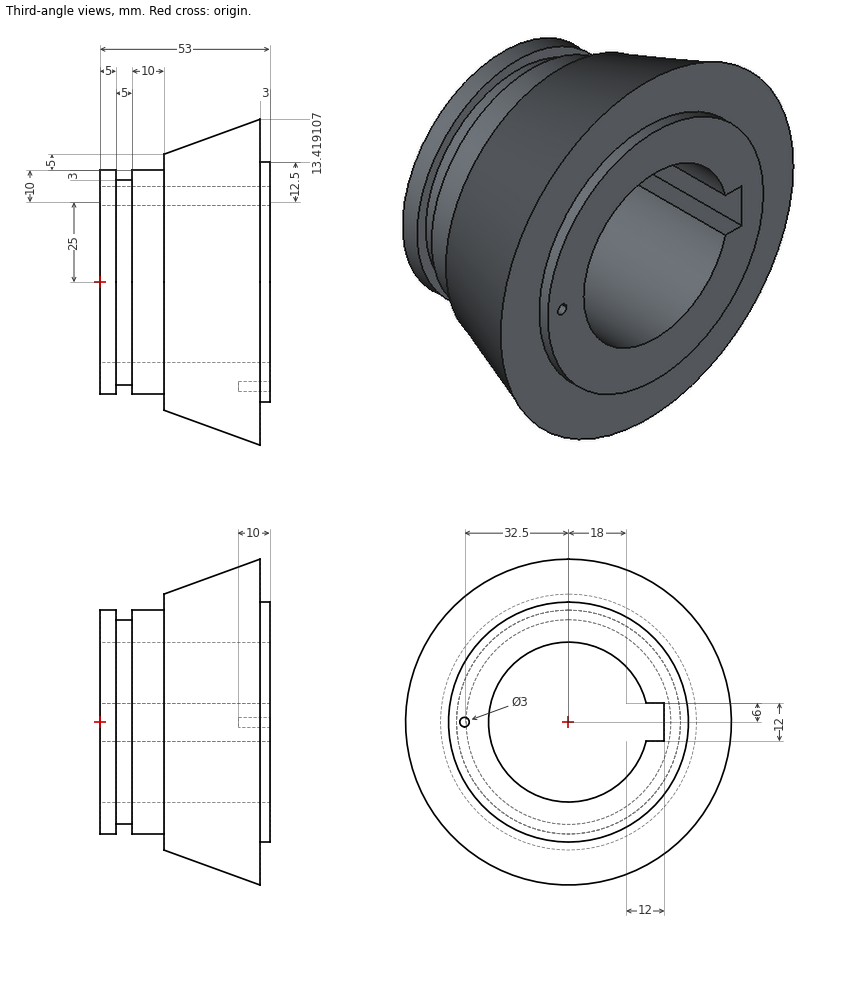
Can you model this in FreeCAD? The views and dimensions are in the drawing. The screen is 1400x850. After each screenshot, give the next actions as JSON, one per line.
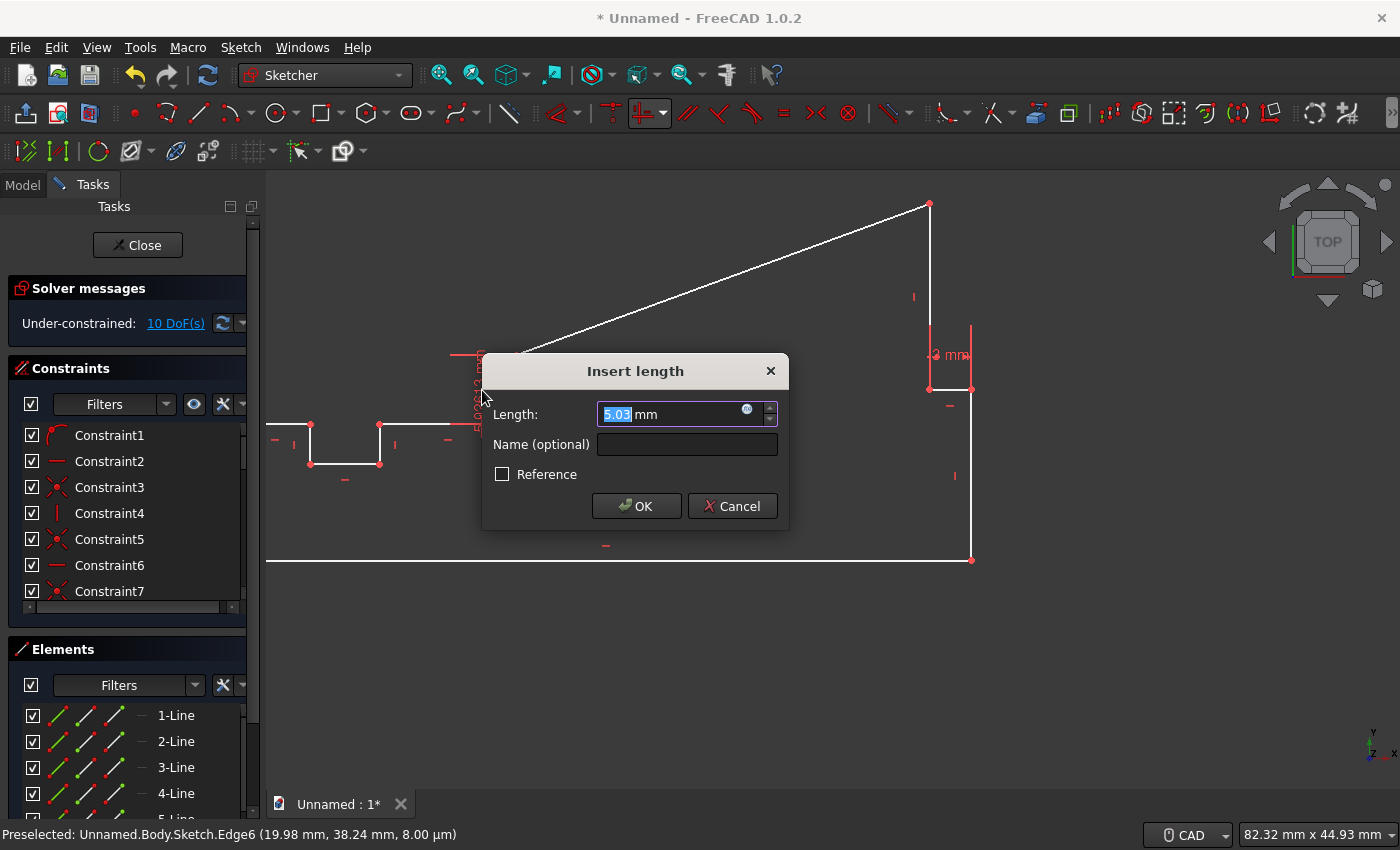
{"action": "type", "text": "5"}
{"action": "key", "text": "Return"}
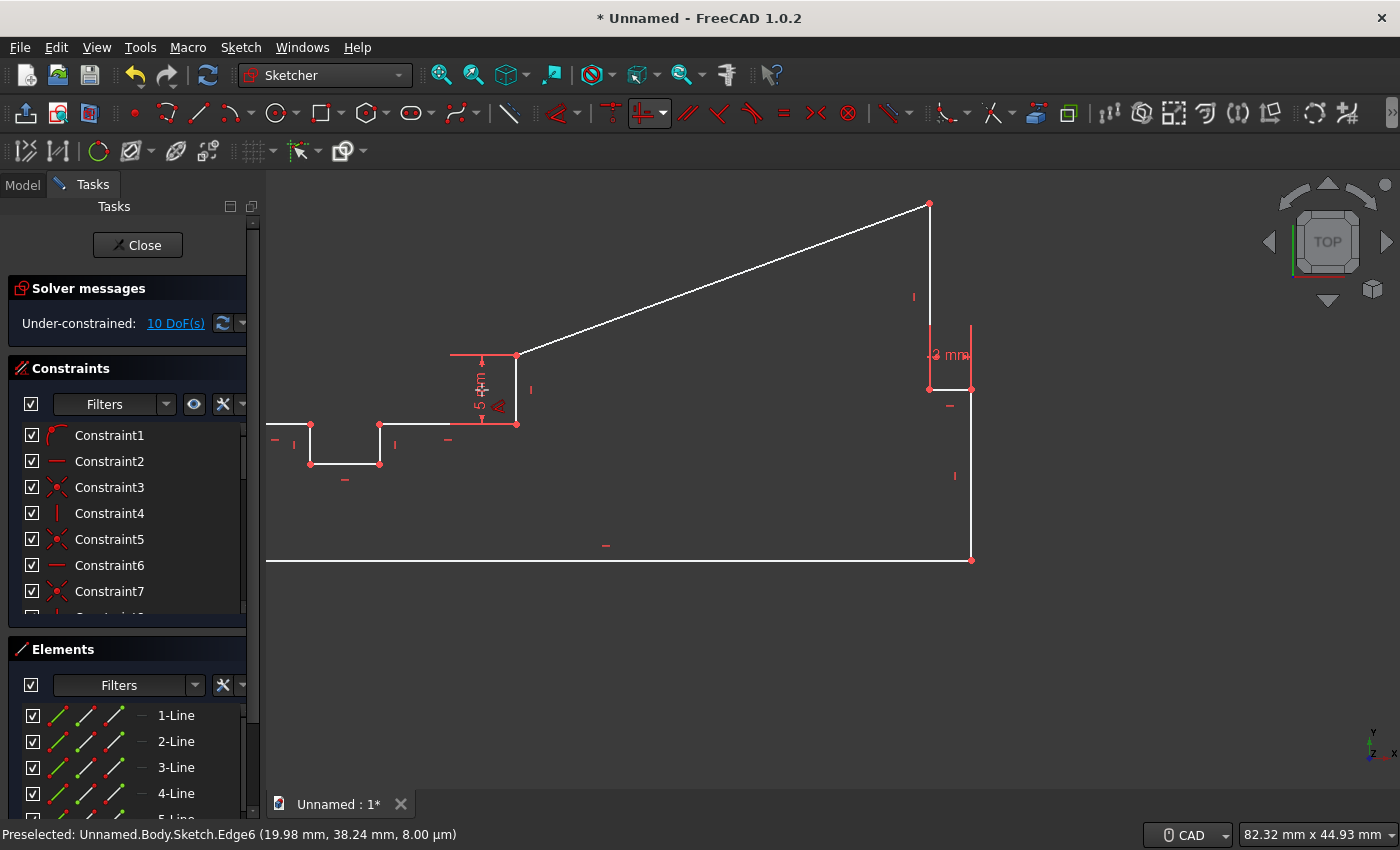
{"action": "left_click", "coordinate": [380, 436]}
{"action": "left_click", "coordinate": [346, 444]}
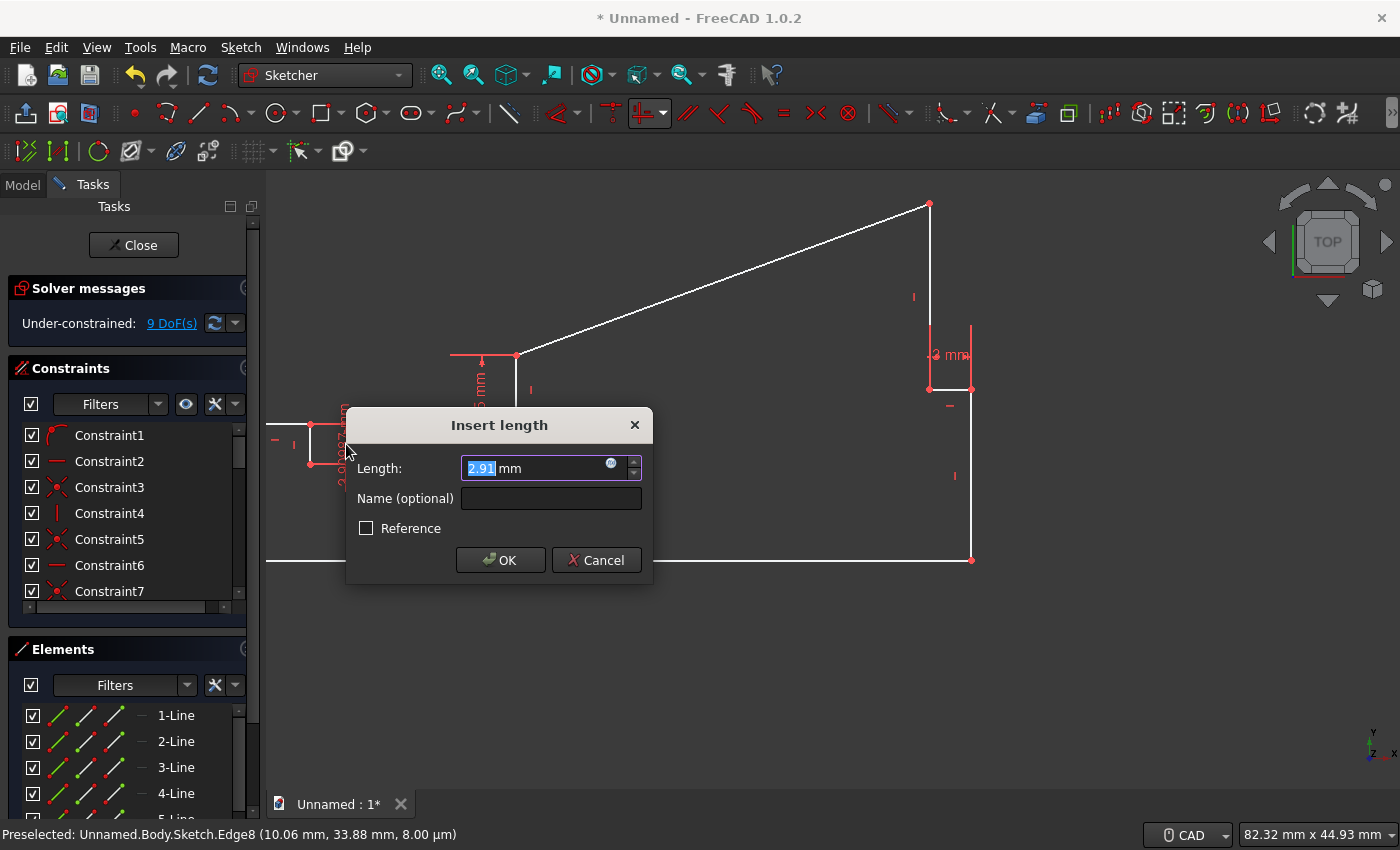
{"action": "type", "text": "3"}
{"action": "key", "text": "Return"}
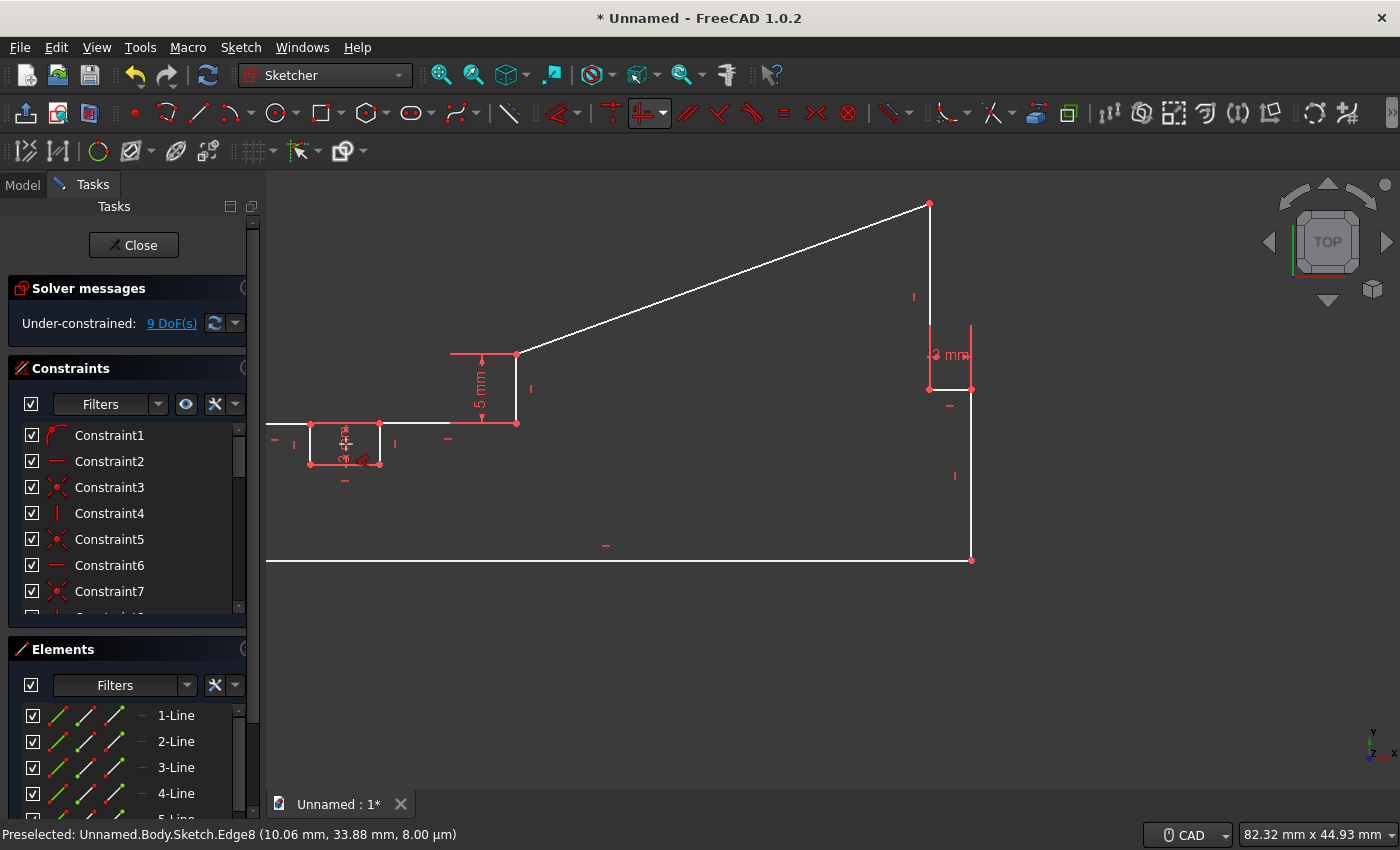
{"action": "left_click", "coordinate": [359, 465]}
{"action": "left_click", "coordinate": [345, 499]}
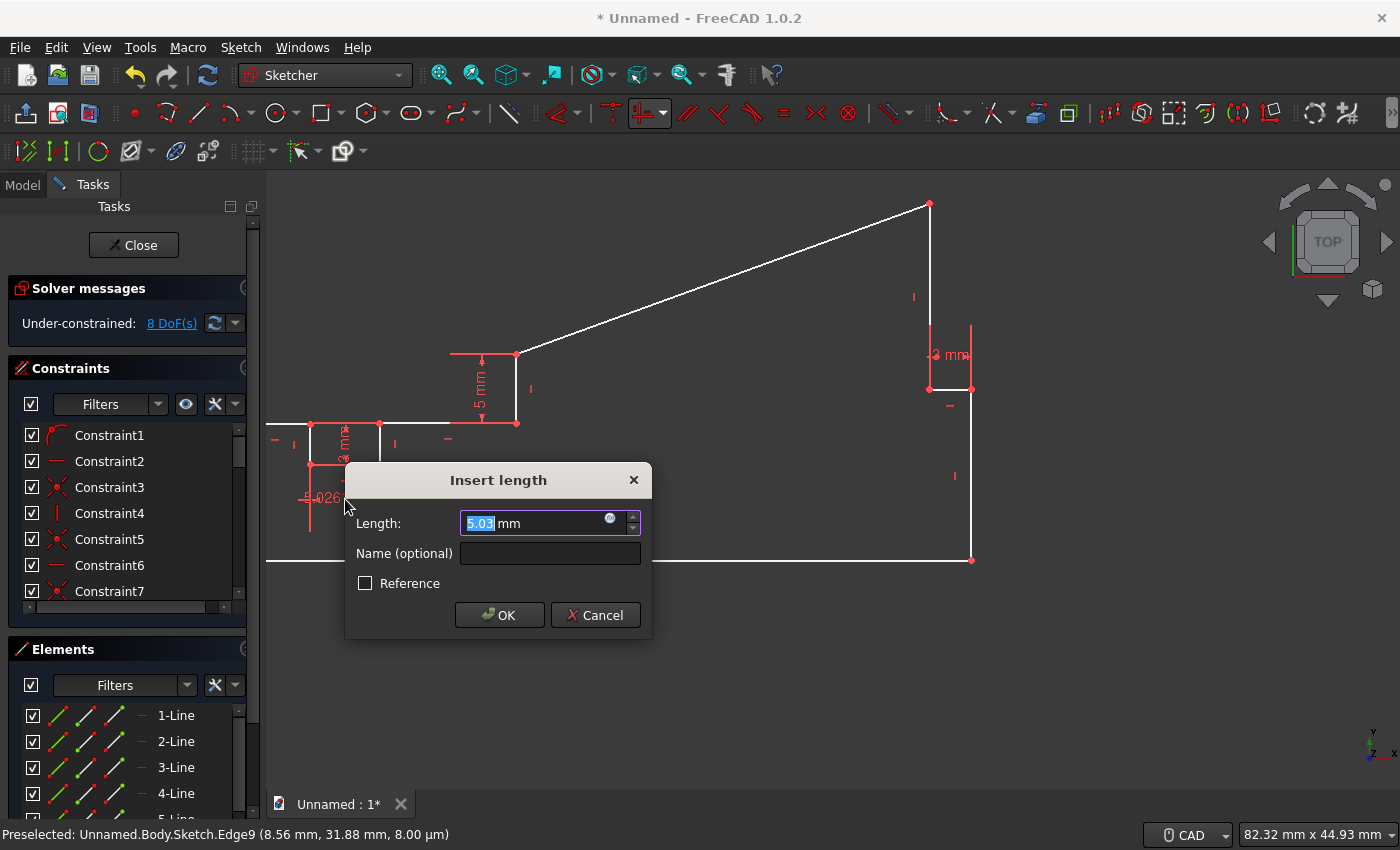
{"action": "type", "text": "5"}
{"action": "key", "text": "Return"}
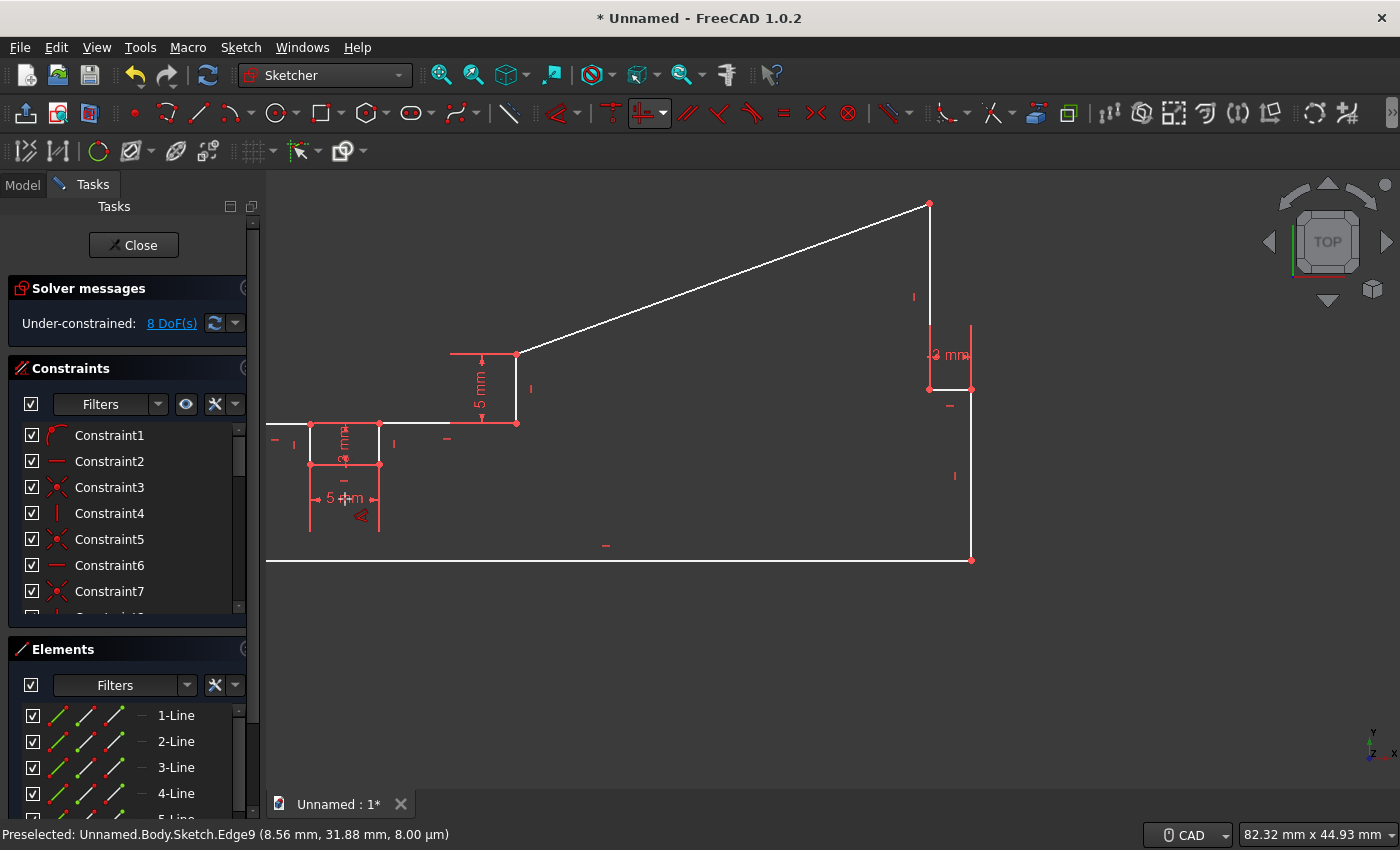
{"action": "left_click", "coordinate": [310, 452]}
{"action": "left_click", "coordinate": [416, 444]}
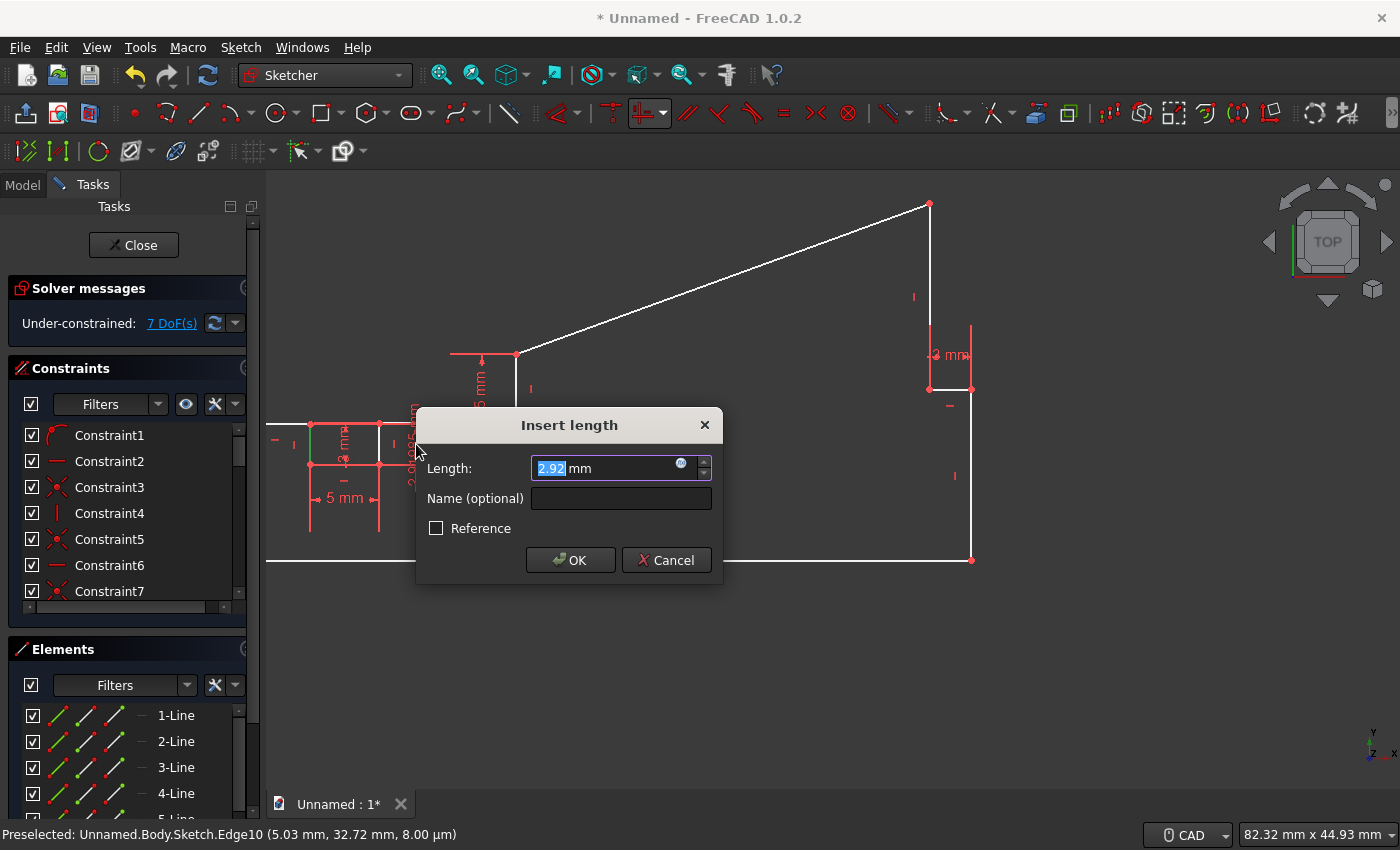
{"action": "type", "text": "3"}
{"action": "key", "text": "Return"}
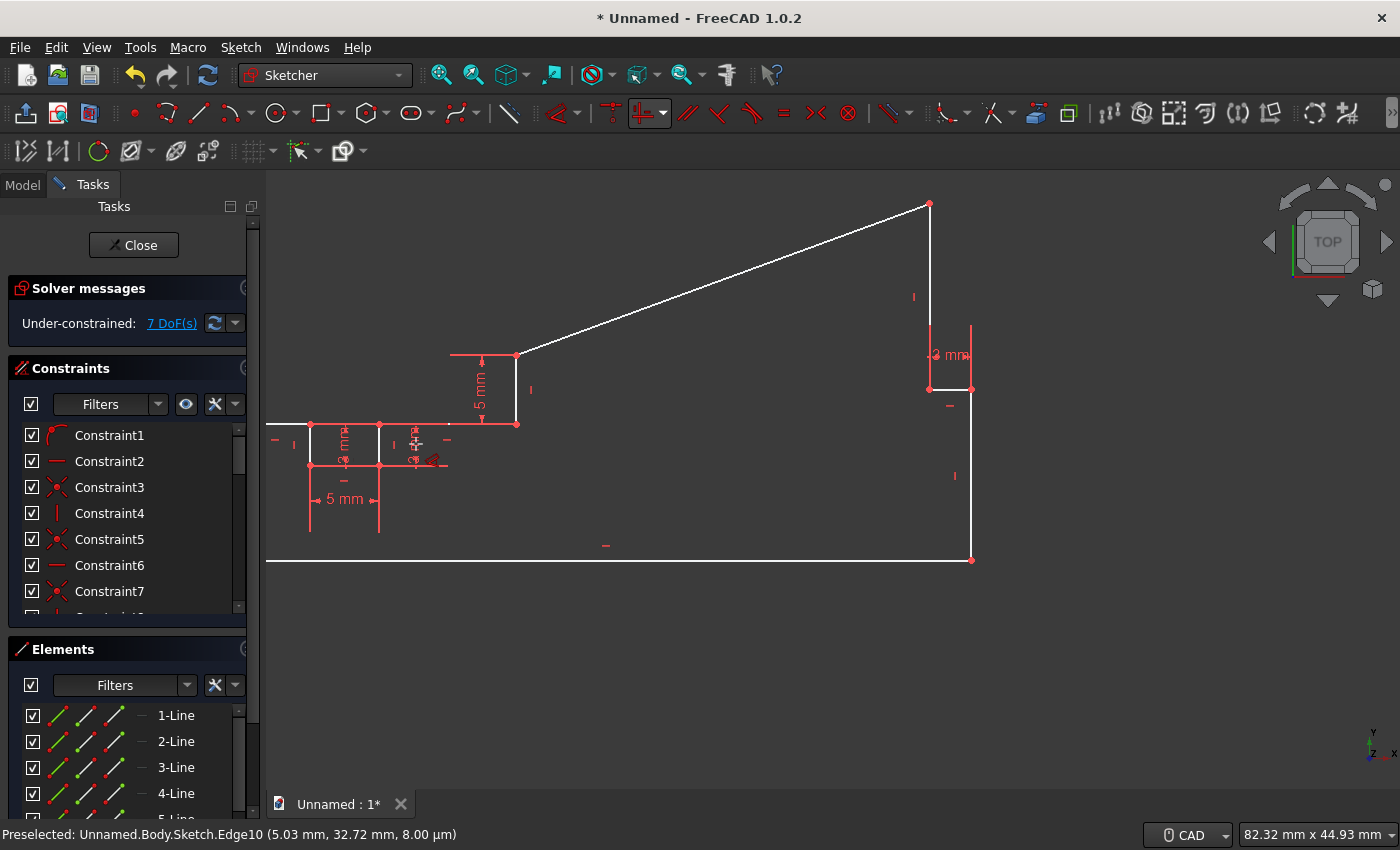
{"action": "left_click", "coordinate": [297, 424]}
{"action": "left_click", "coordinate": [302, 390]}